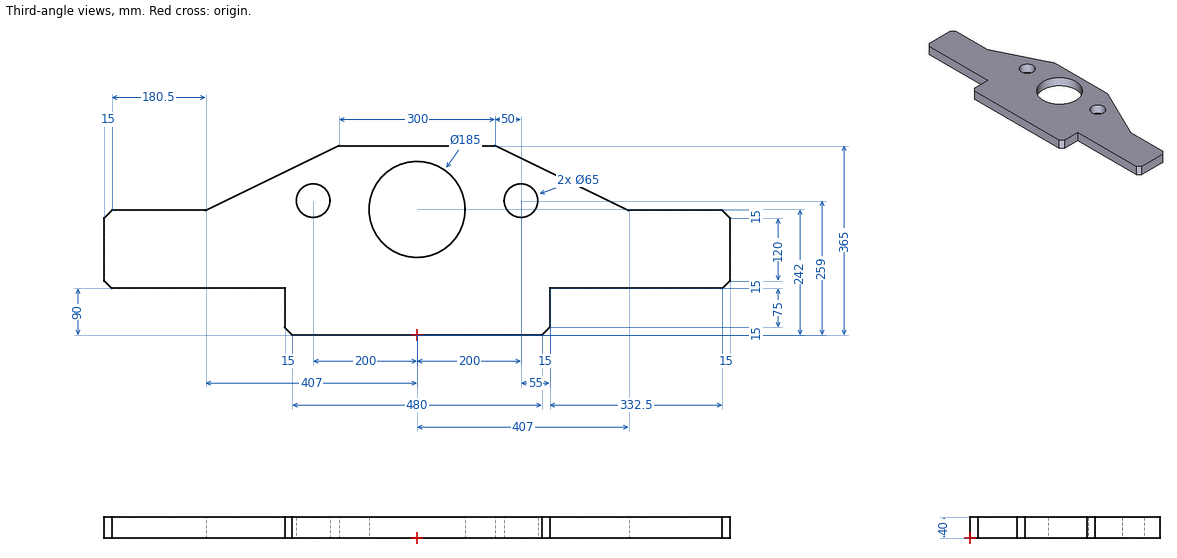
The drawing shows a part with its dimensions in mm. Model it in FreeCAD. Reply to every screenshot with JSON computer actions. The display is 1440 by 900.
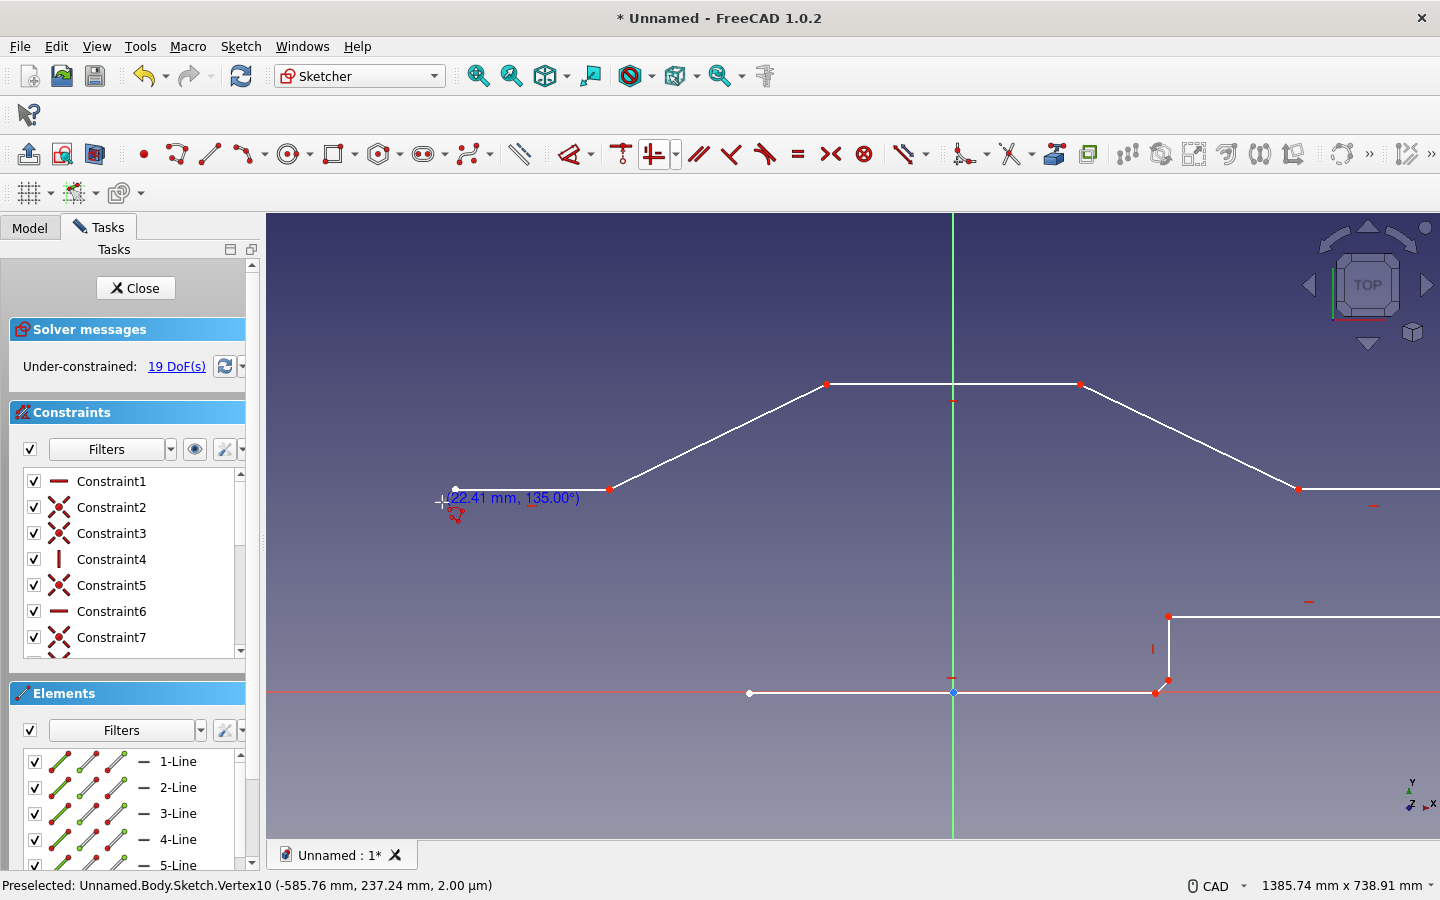
{"action": "left_click", "coordinate": [443, 502]}
{"action": "left_click", "coordinate": [443, 603]}
{"action": "left_click", "coordinate": [455, 616]}
{"action": "left_click", "coordinate": [737, 616]}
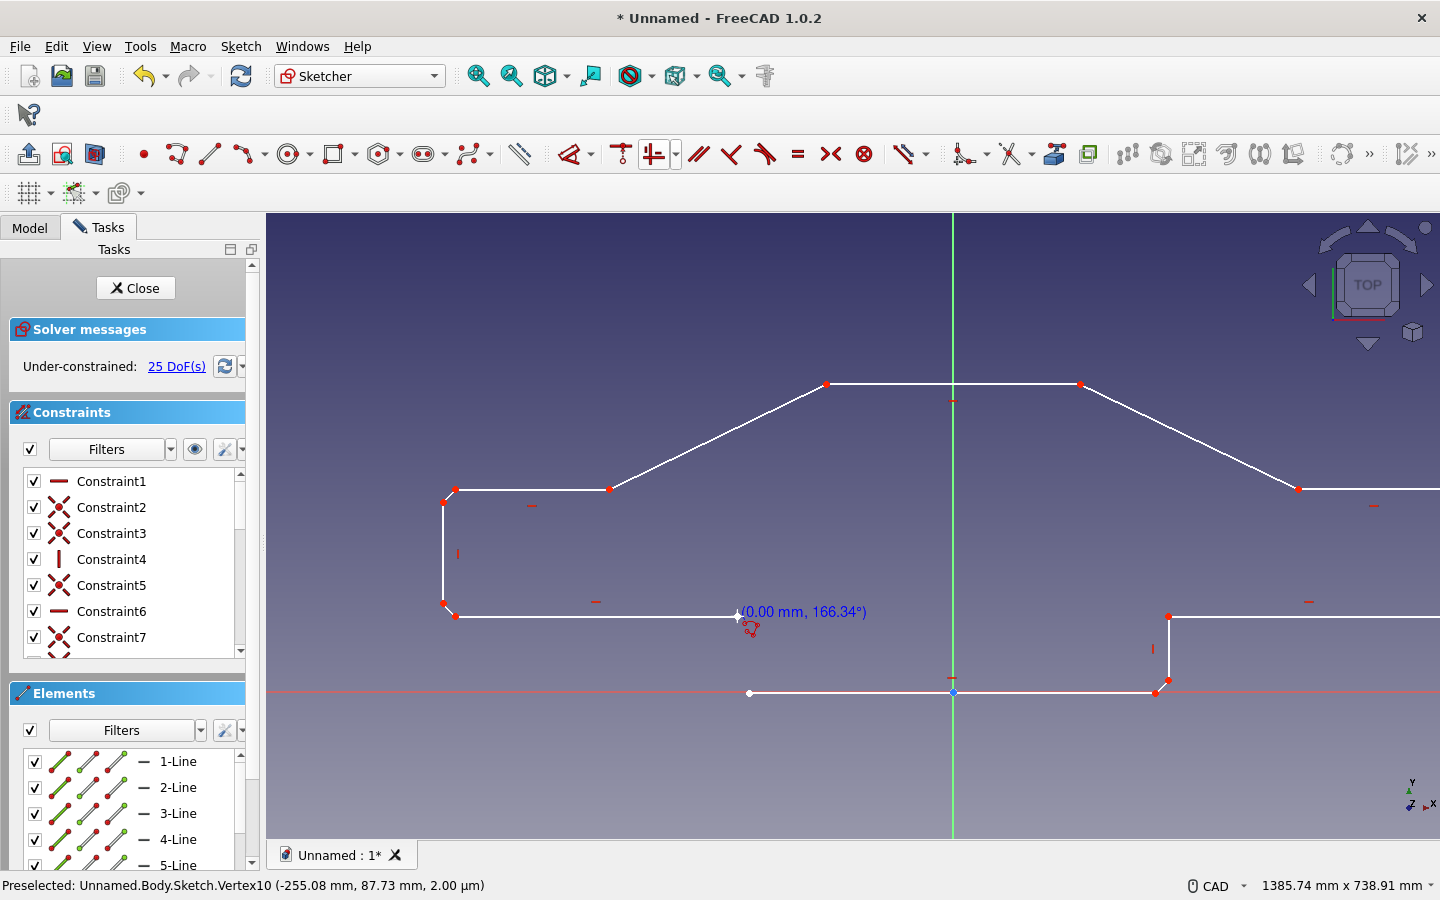
{"action": "scroll", "coordinate": [737, 680], "scroll_direction": "up", "scroll_amount": 2}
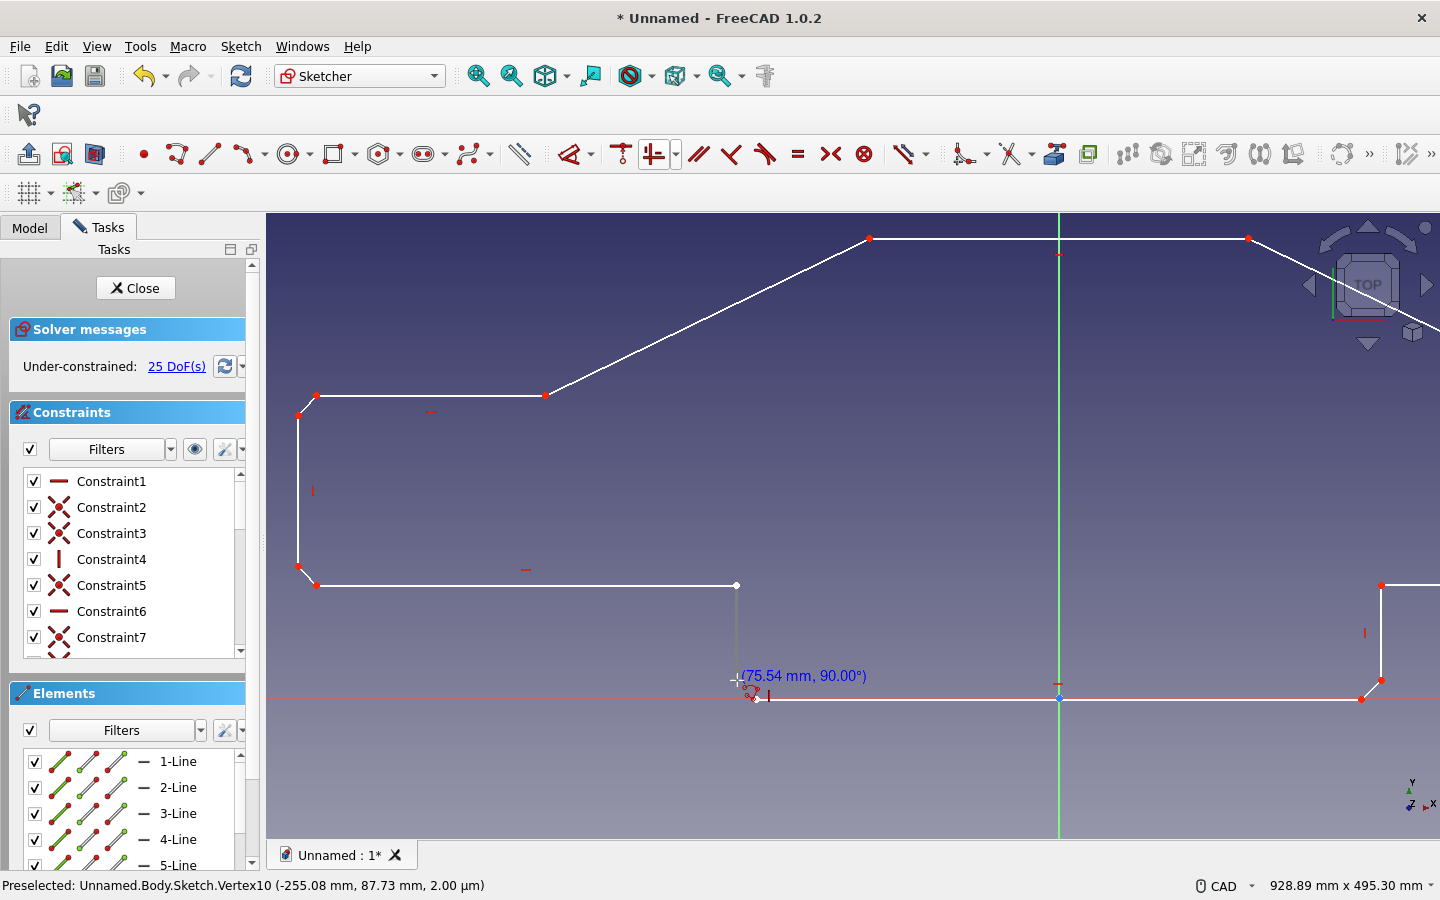
{"action": "left_click", "coordinate": [737, 679]}
{"action": "left_click", "coordinate": [756, 700]}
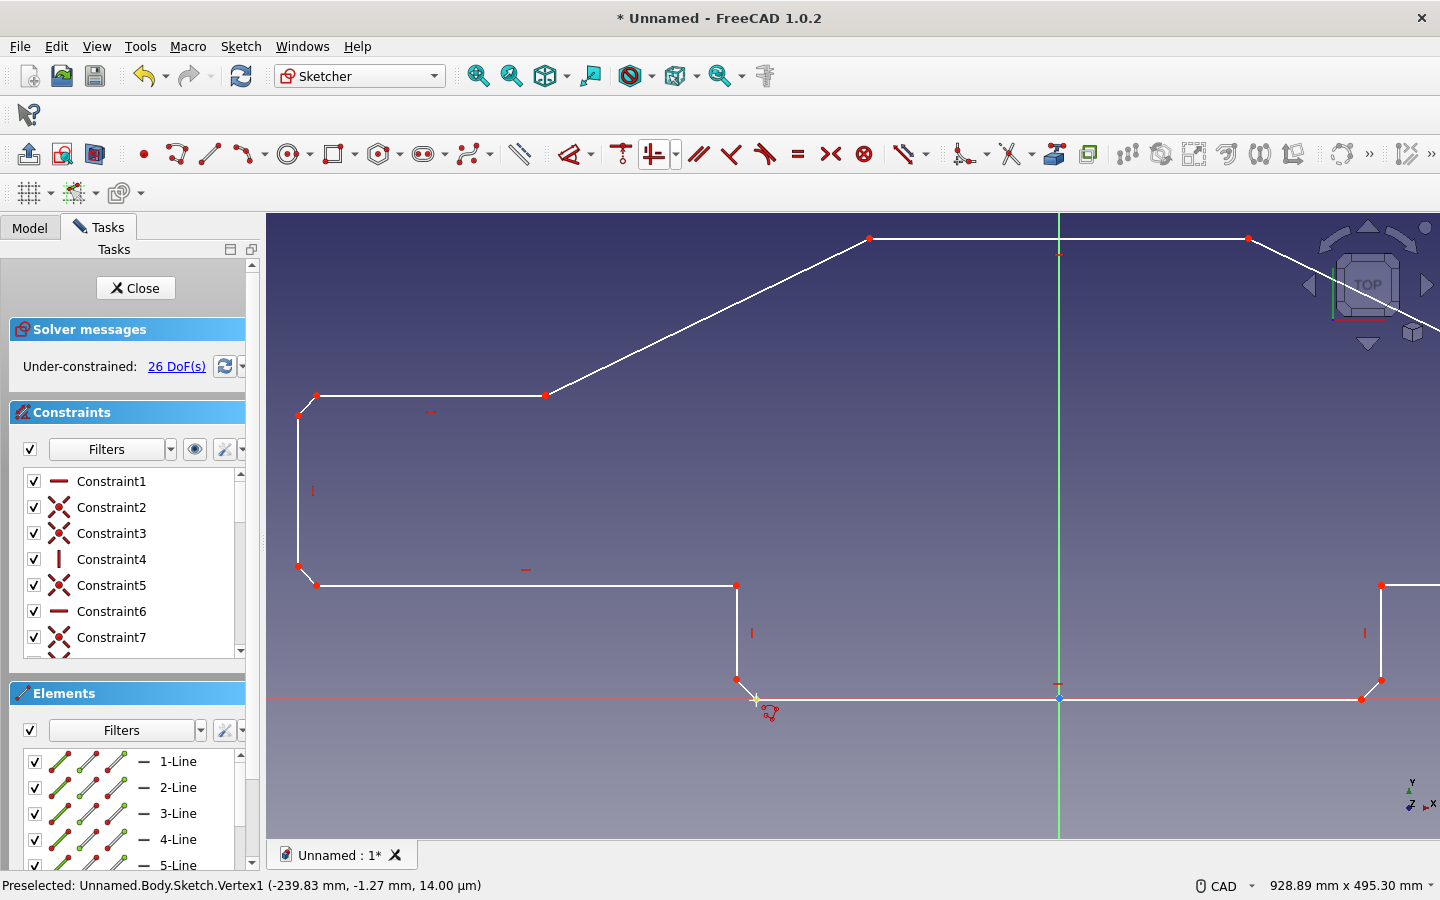
{"action": "left_click", "coordinate": [288, 154]}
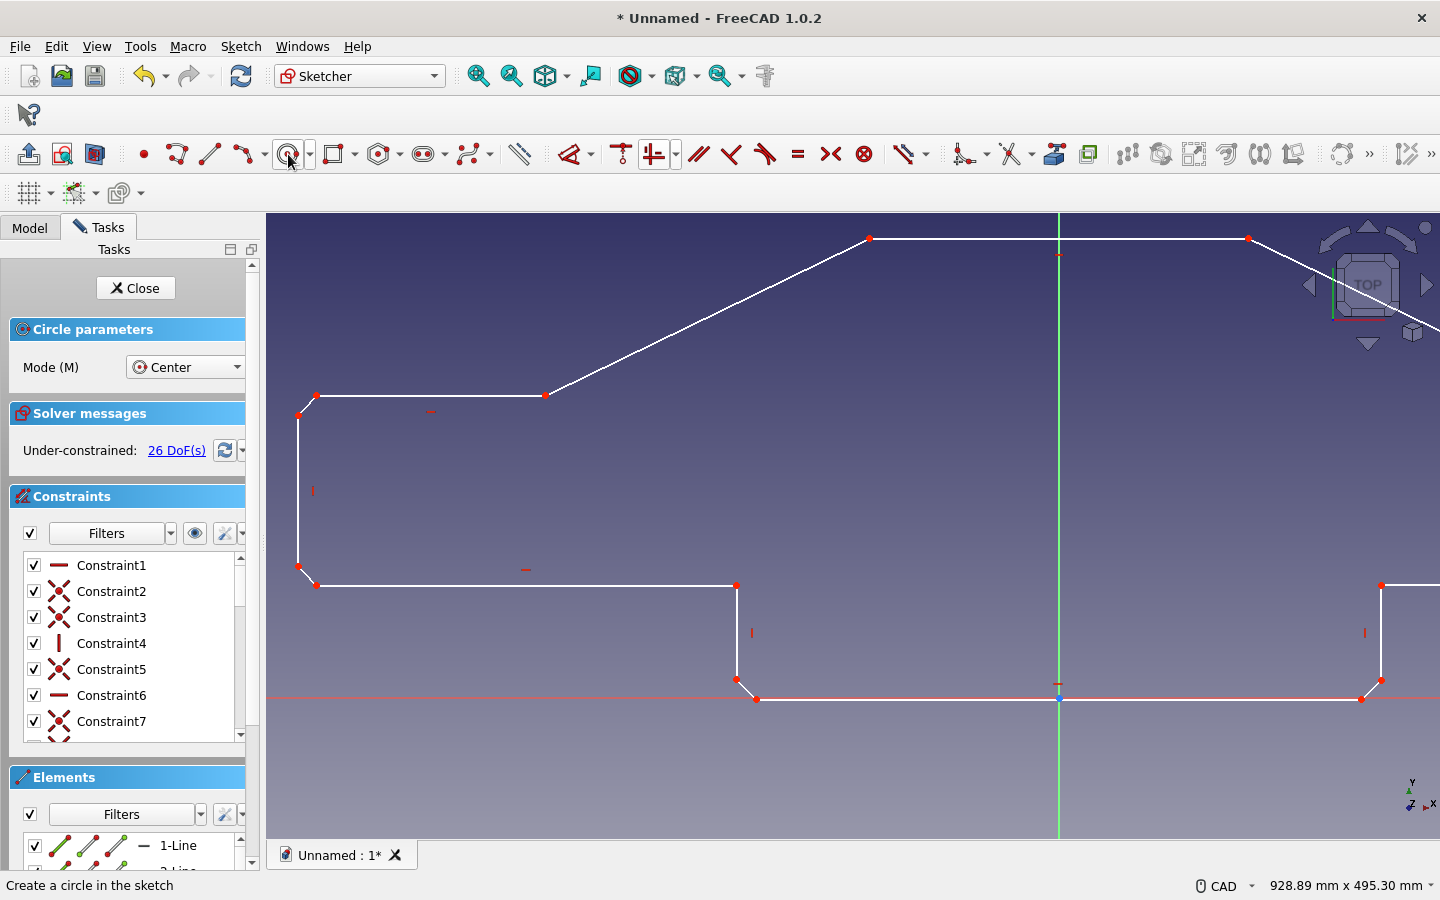
{"action": "scroll", "coordinate": [560, 574], "scroll_direction": "down", "scroll_amount": 4}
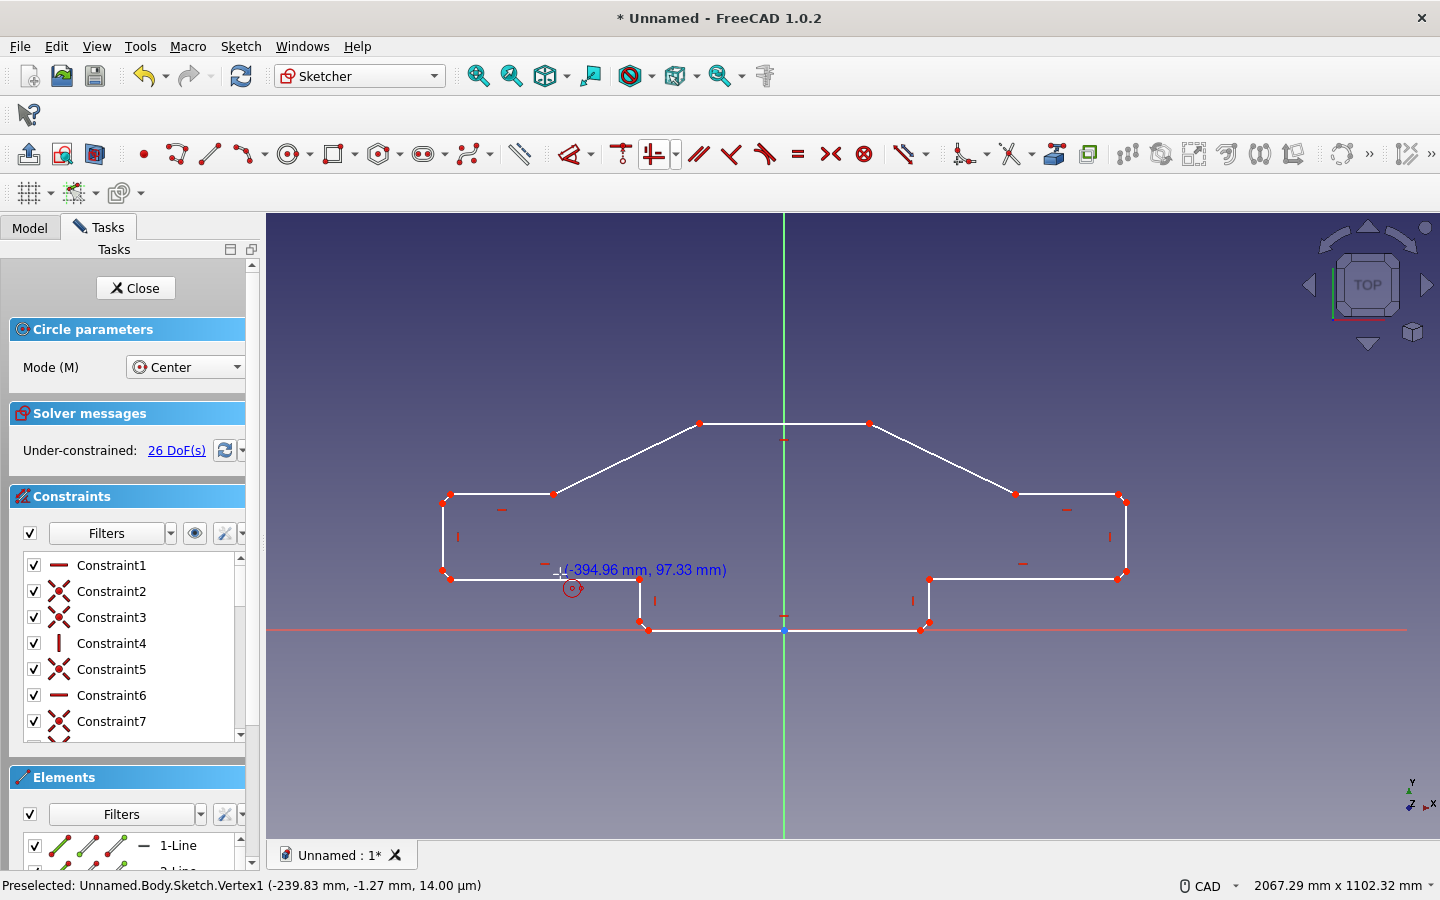
{"action": "scroll", "coordinate": [898, 483], "scroll_direction": "up", "scroll_amount": 2}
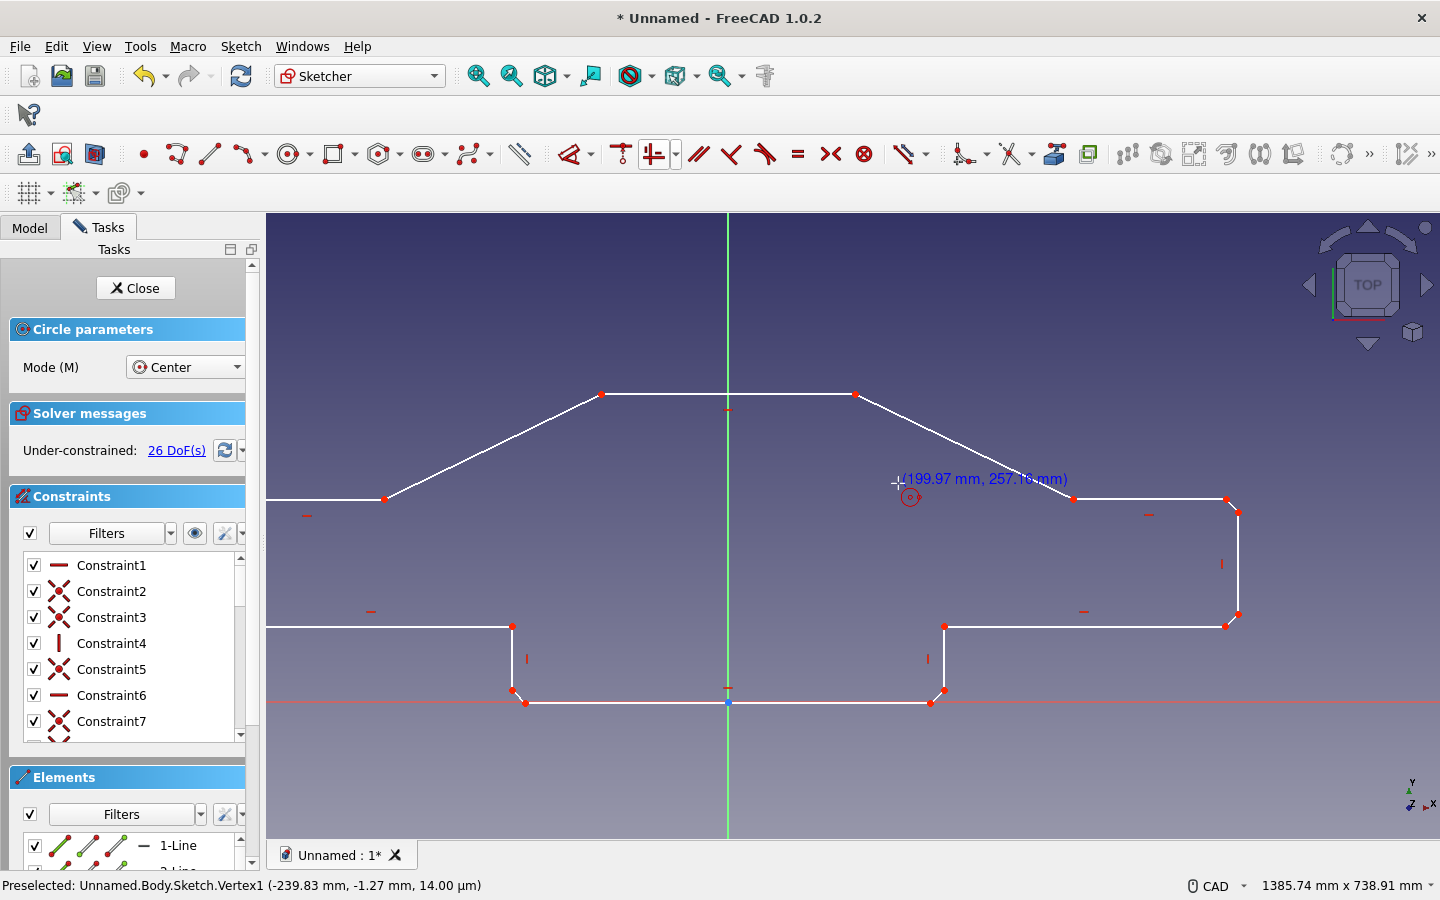
{"action": "left_click", "coordinate": [898, 483]}
{"action": "left_click", "coordinate": [917, 463]}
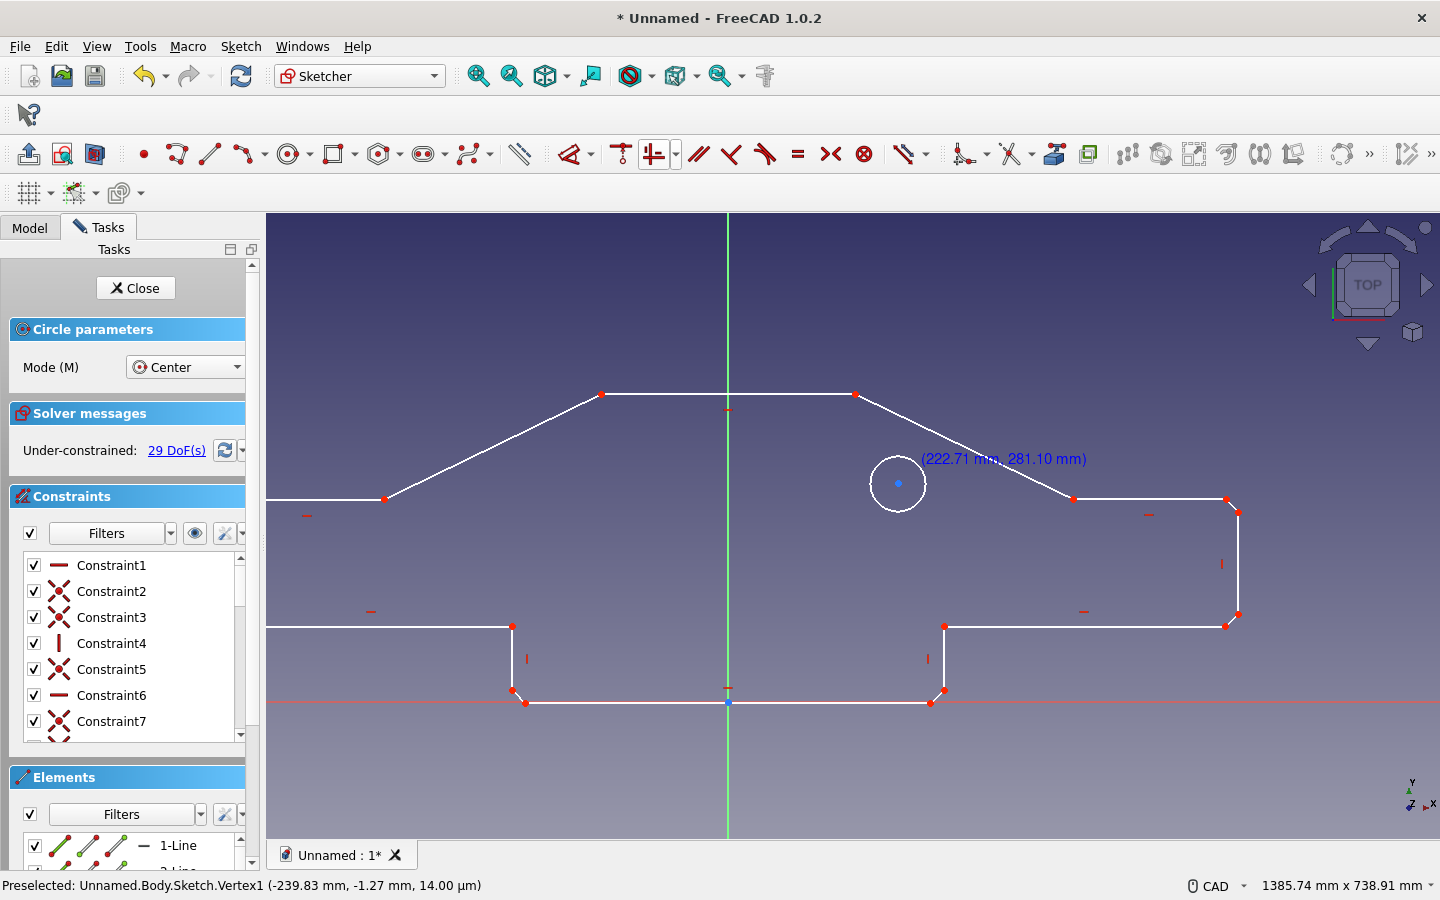
{"action": "left_click", "coordinate": [728, 497]}
{"action": "left_click", "coordinate": [784, 442]}